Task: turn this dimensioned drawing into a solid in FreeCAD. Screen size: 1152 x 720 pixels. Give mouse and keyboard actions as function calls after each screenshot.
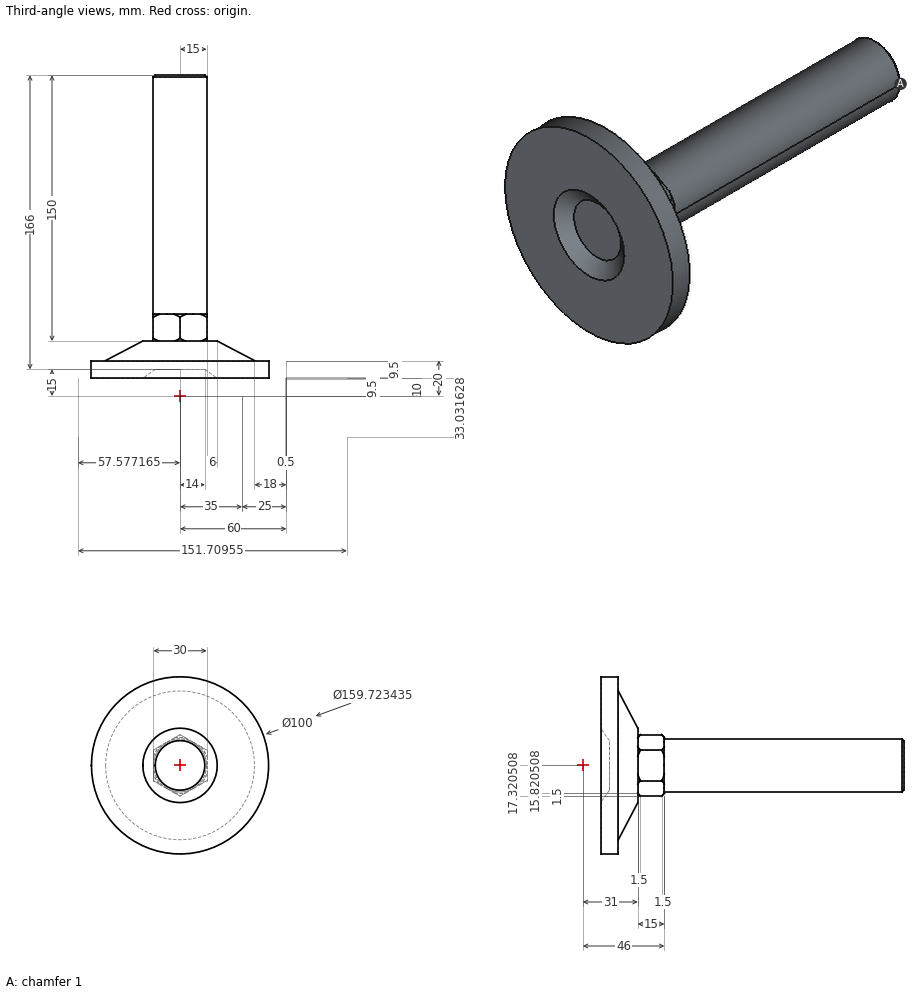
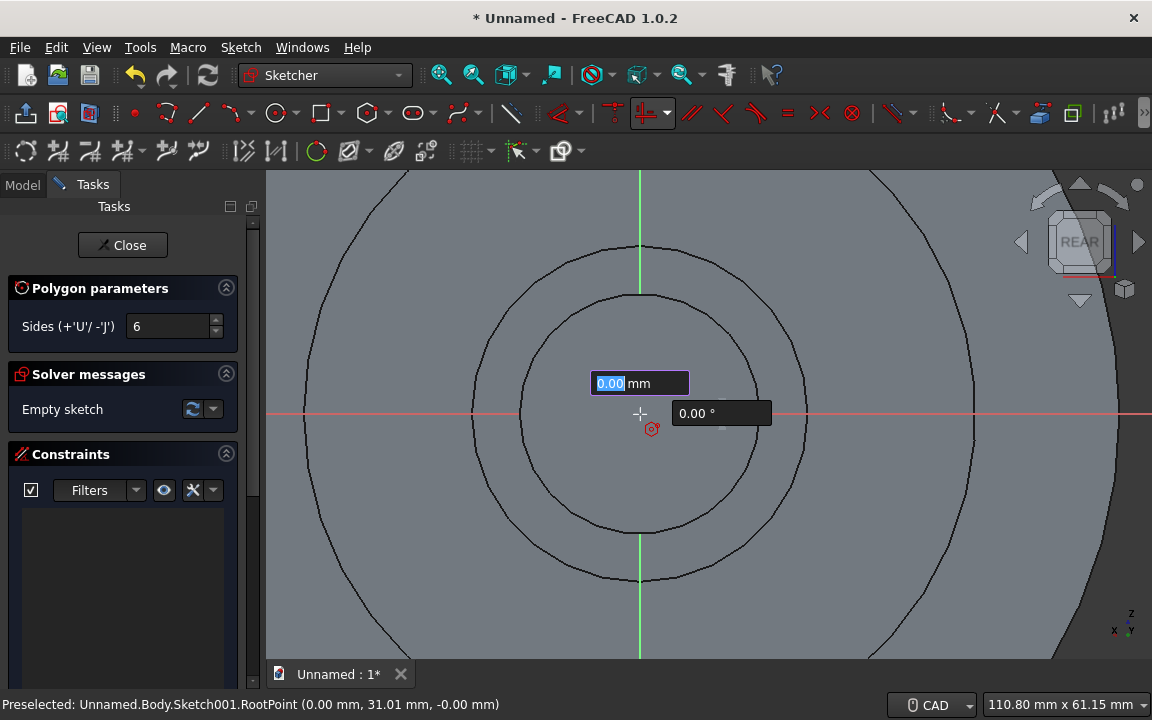
click(640, 552)
right_click(640, 552)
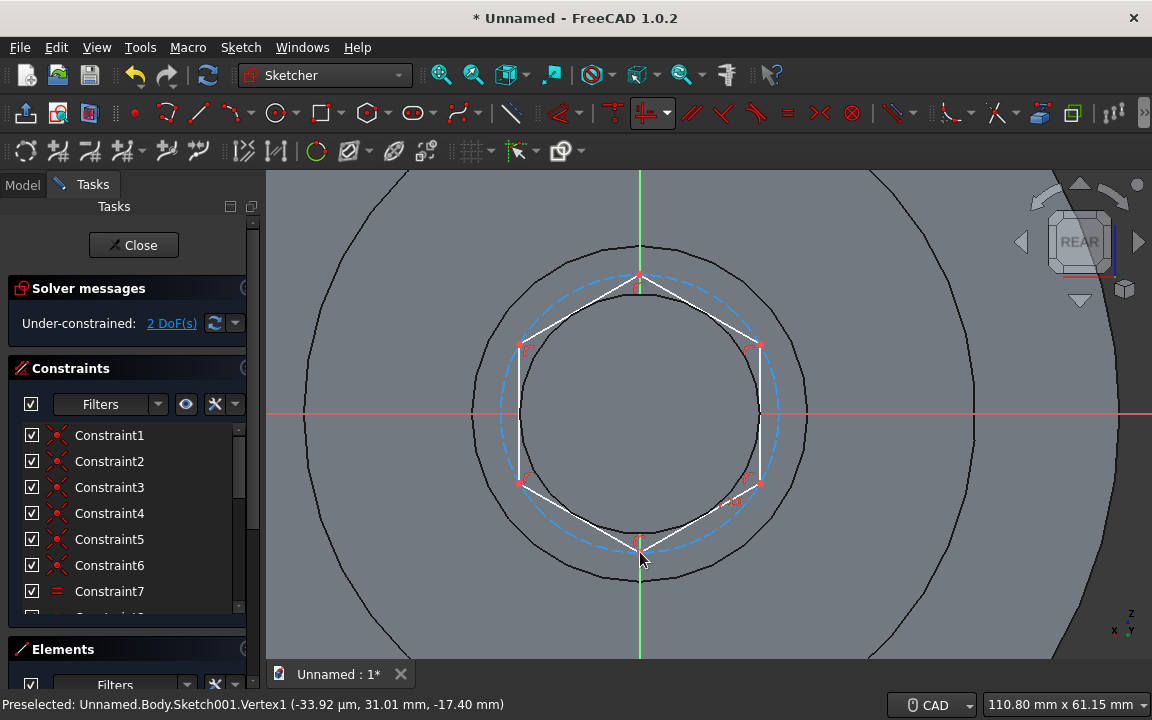
click(760, 441)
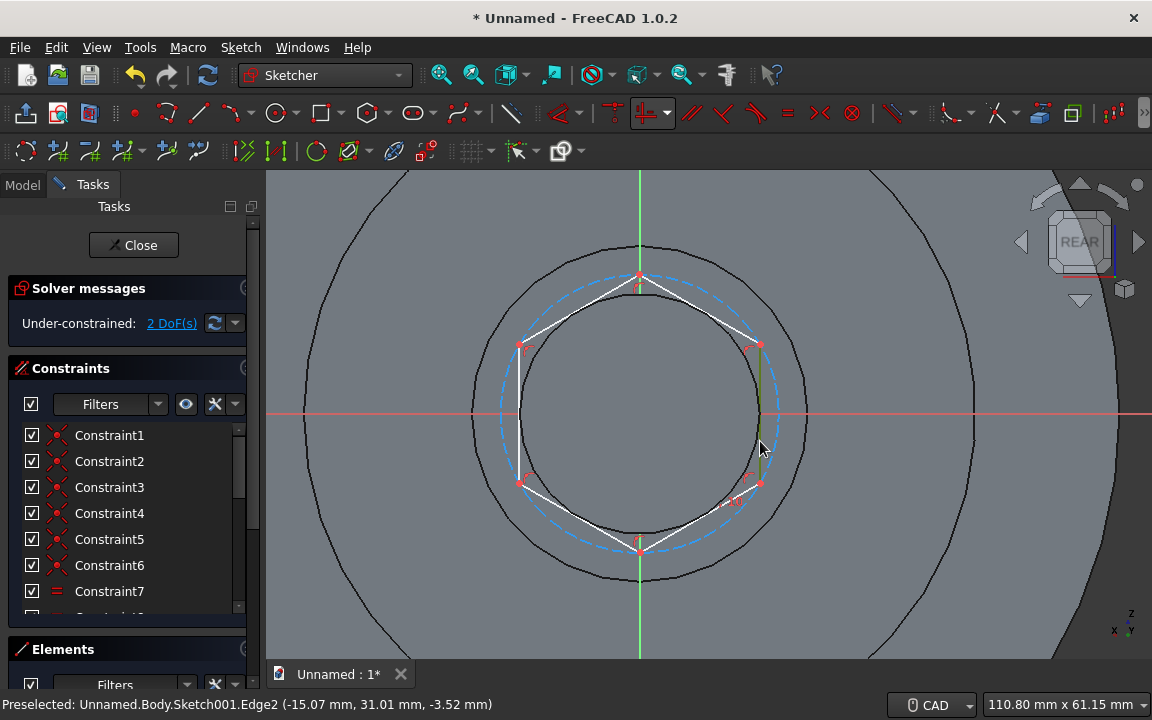
key(v)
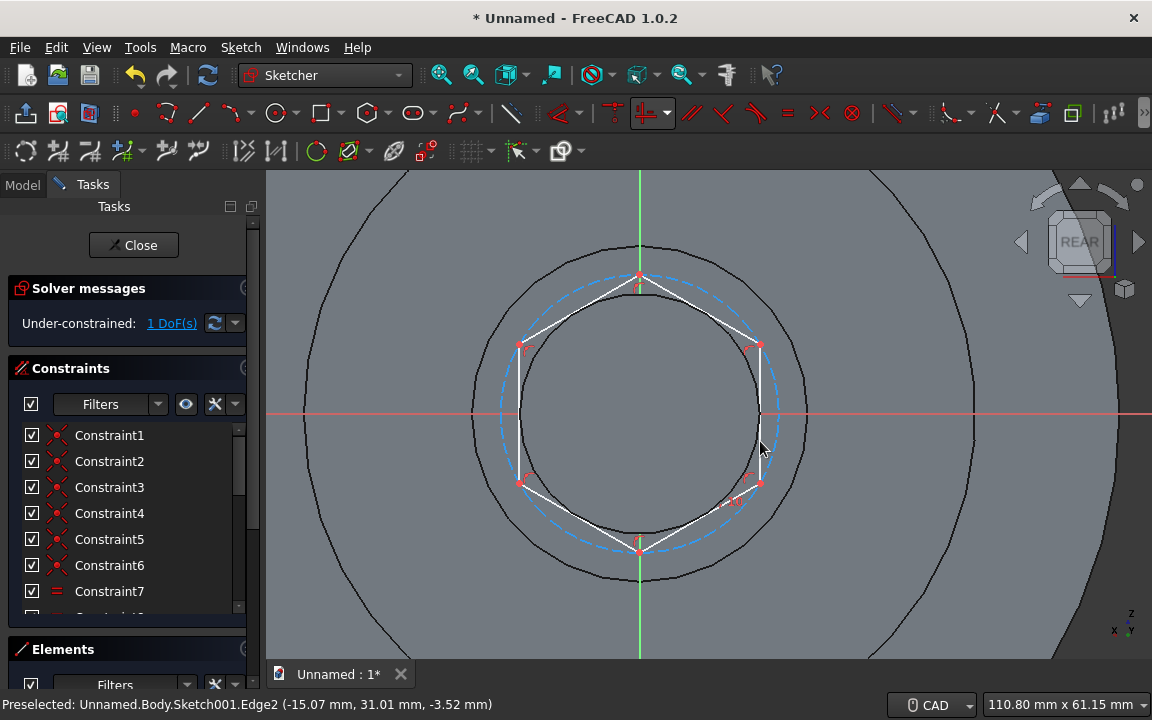
click(558, 114)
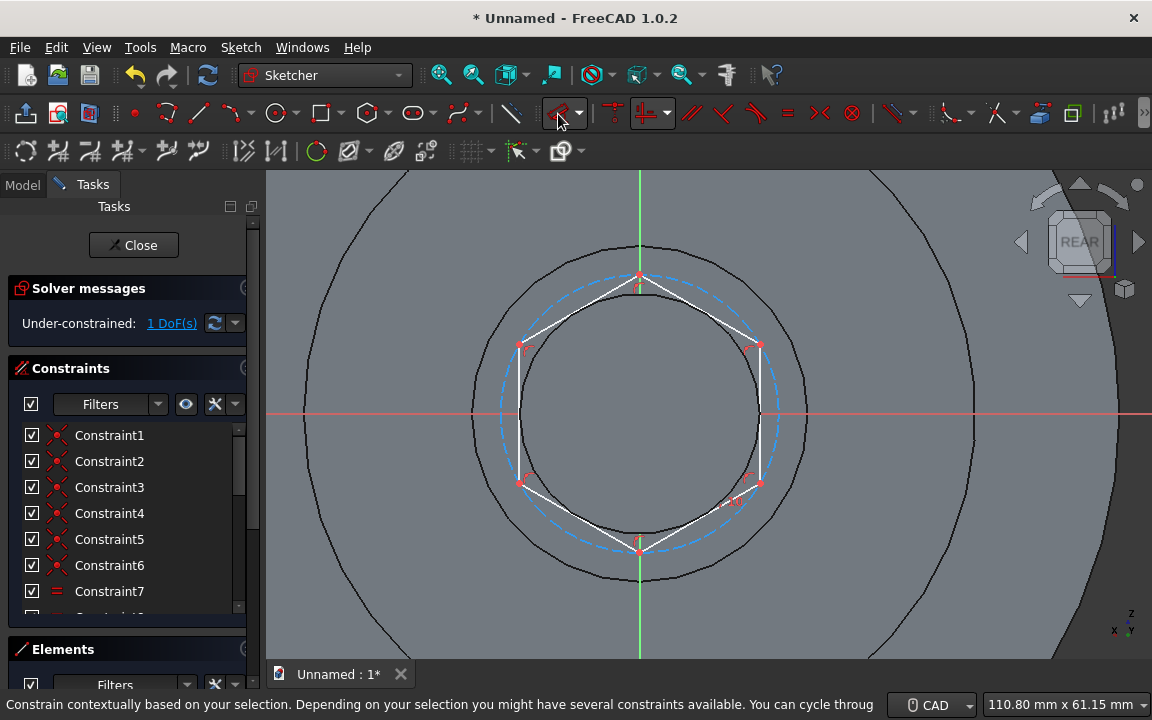
click(519, 344)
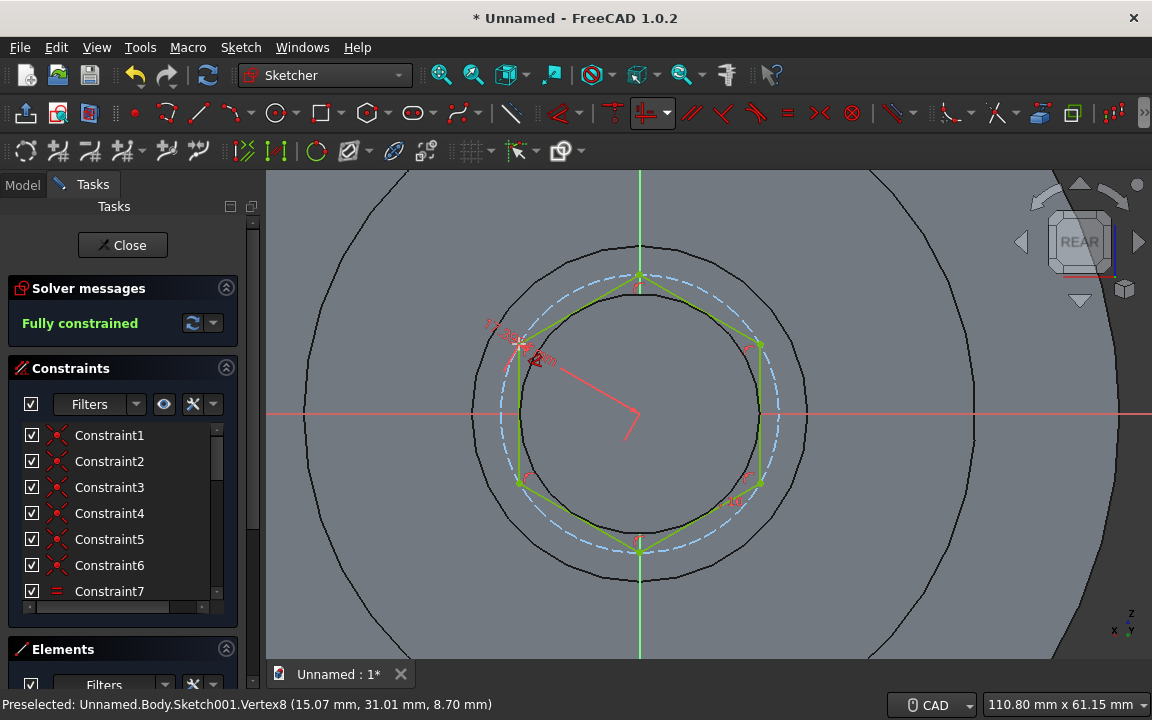
click(760, 483)
click(555, 286)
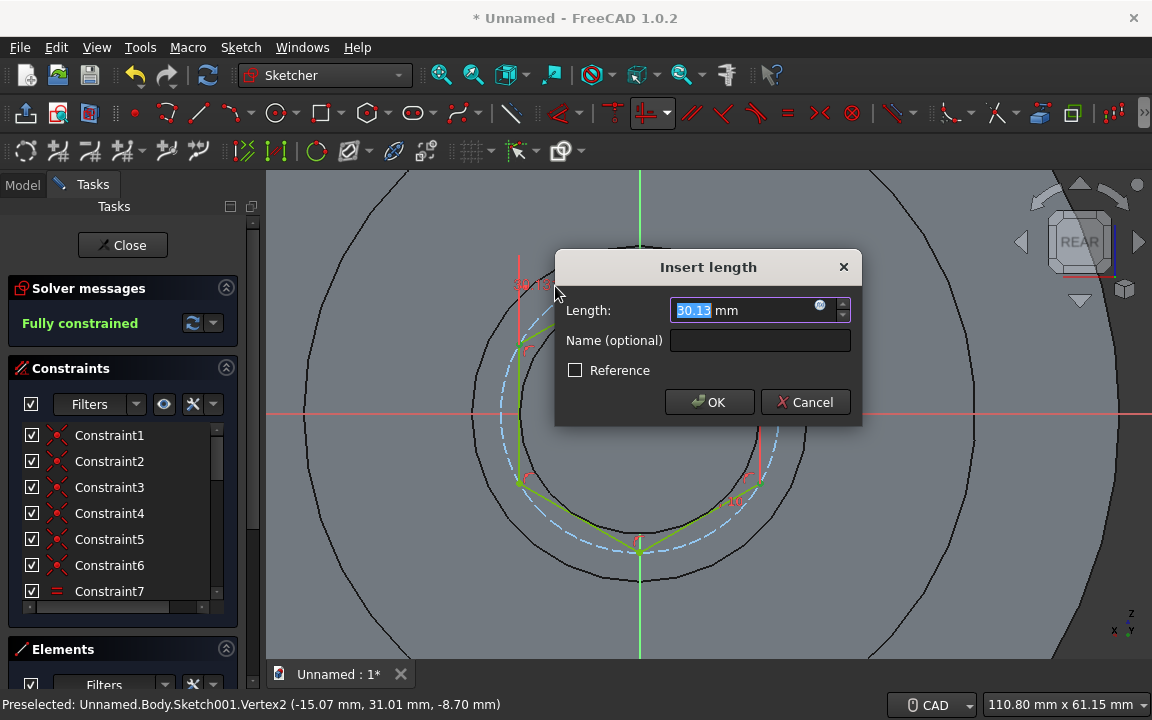
text(30)
key(Return)
key(Escape)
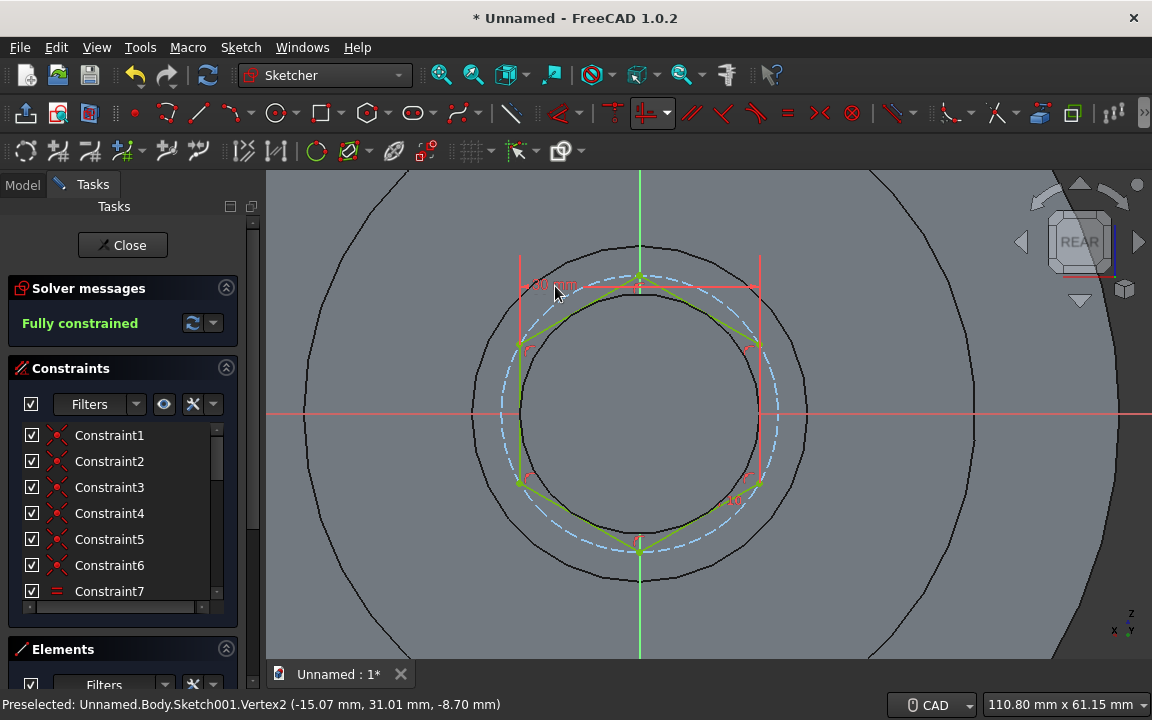
click(123, 245)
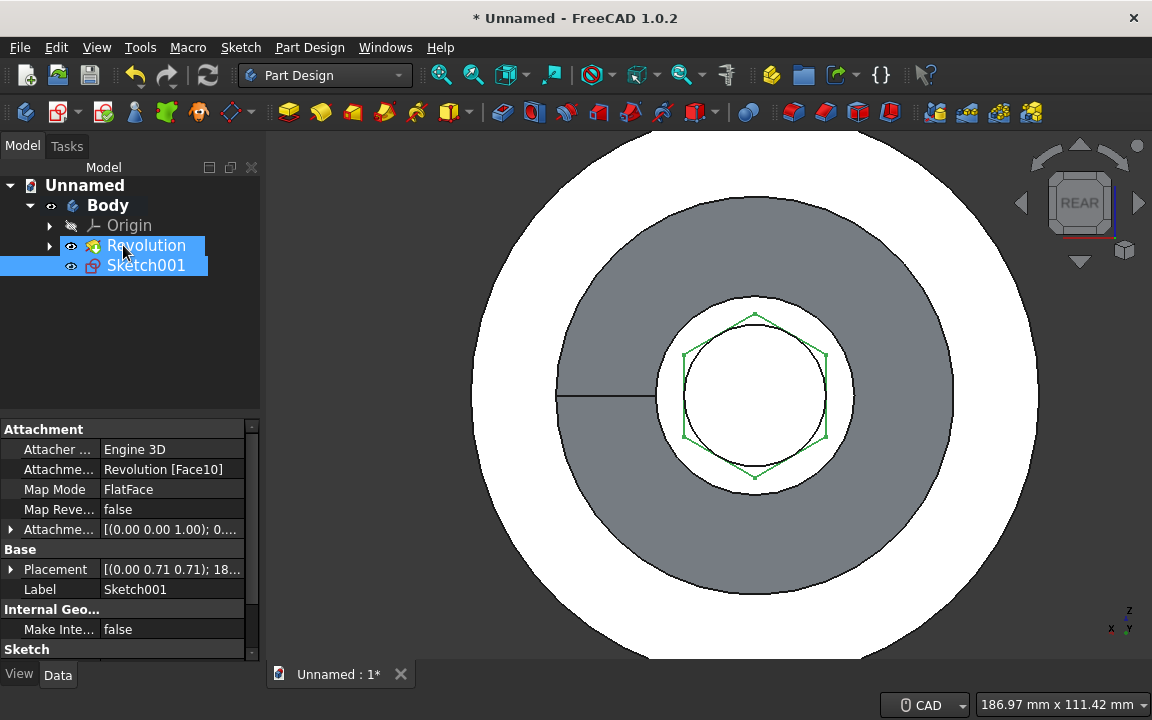
click(290, 112)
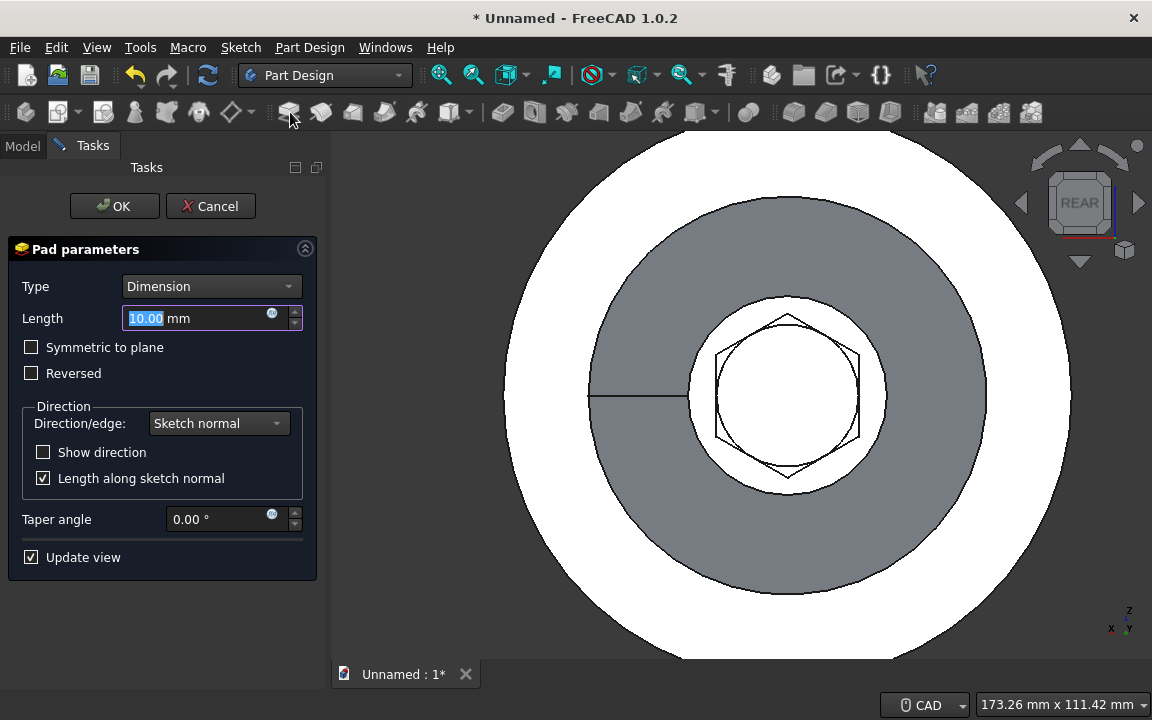
text(15)
key(Tab)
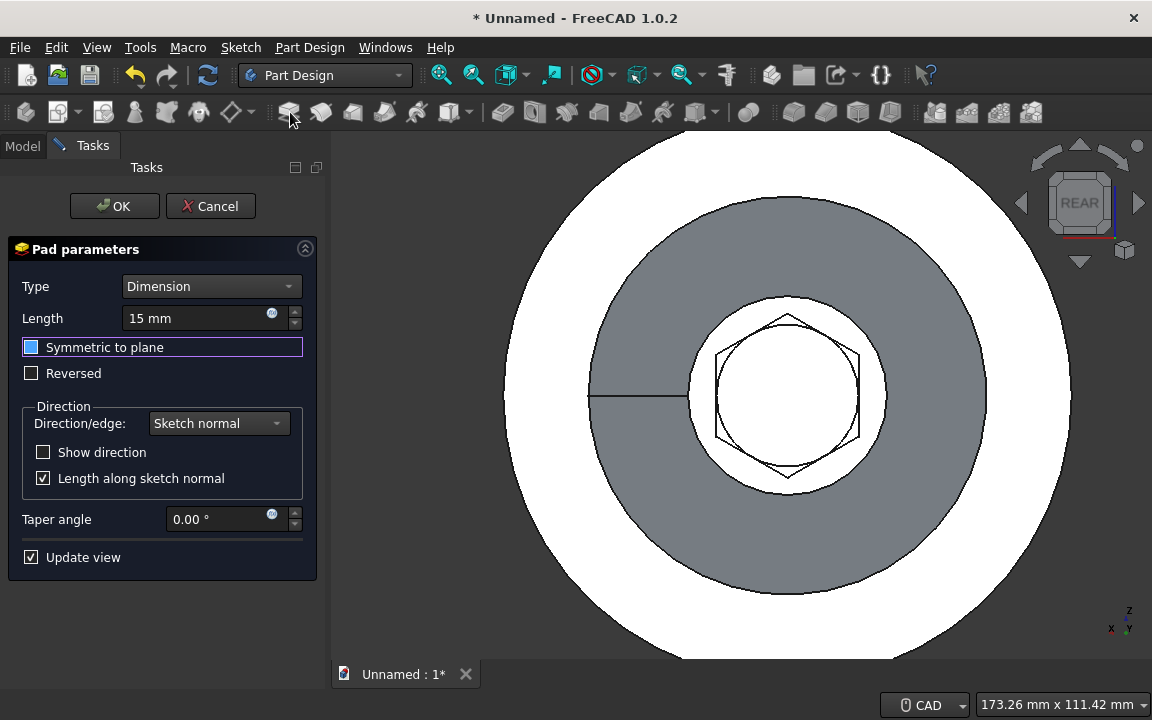
click(115, 206)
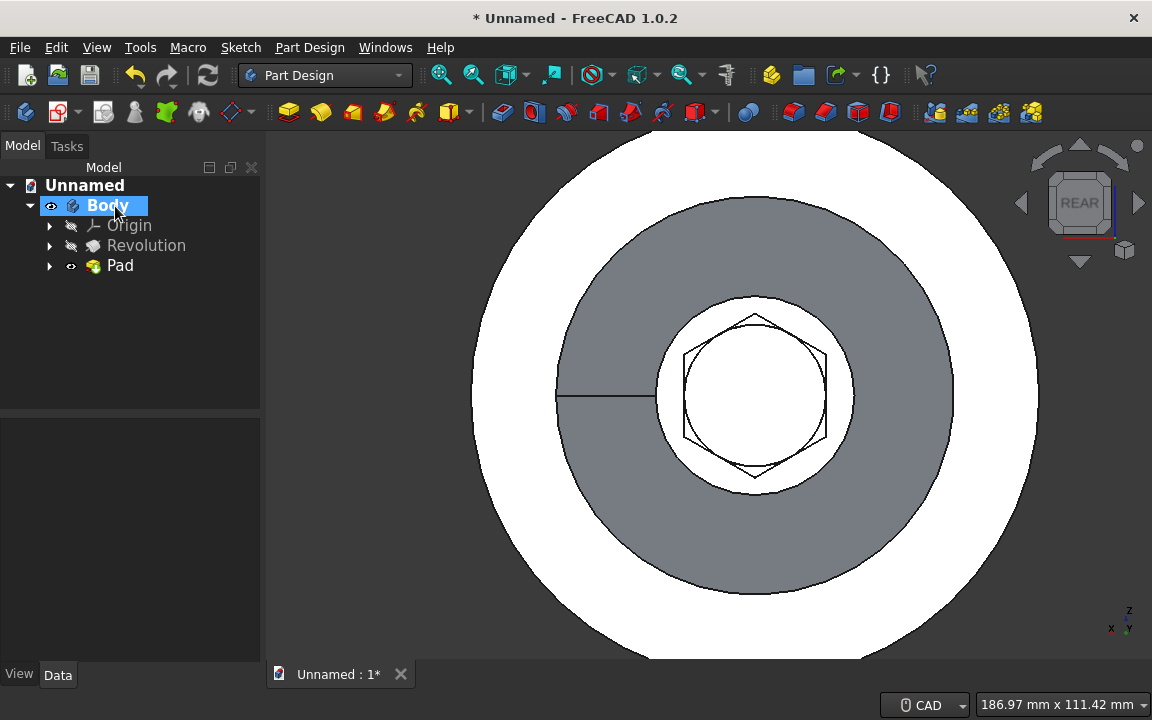
key(v)
key(f)